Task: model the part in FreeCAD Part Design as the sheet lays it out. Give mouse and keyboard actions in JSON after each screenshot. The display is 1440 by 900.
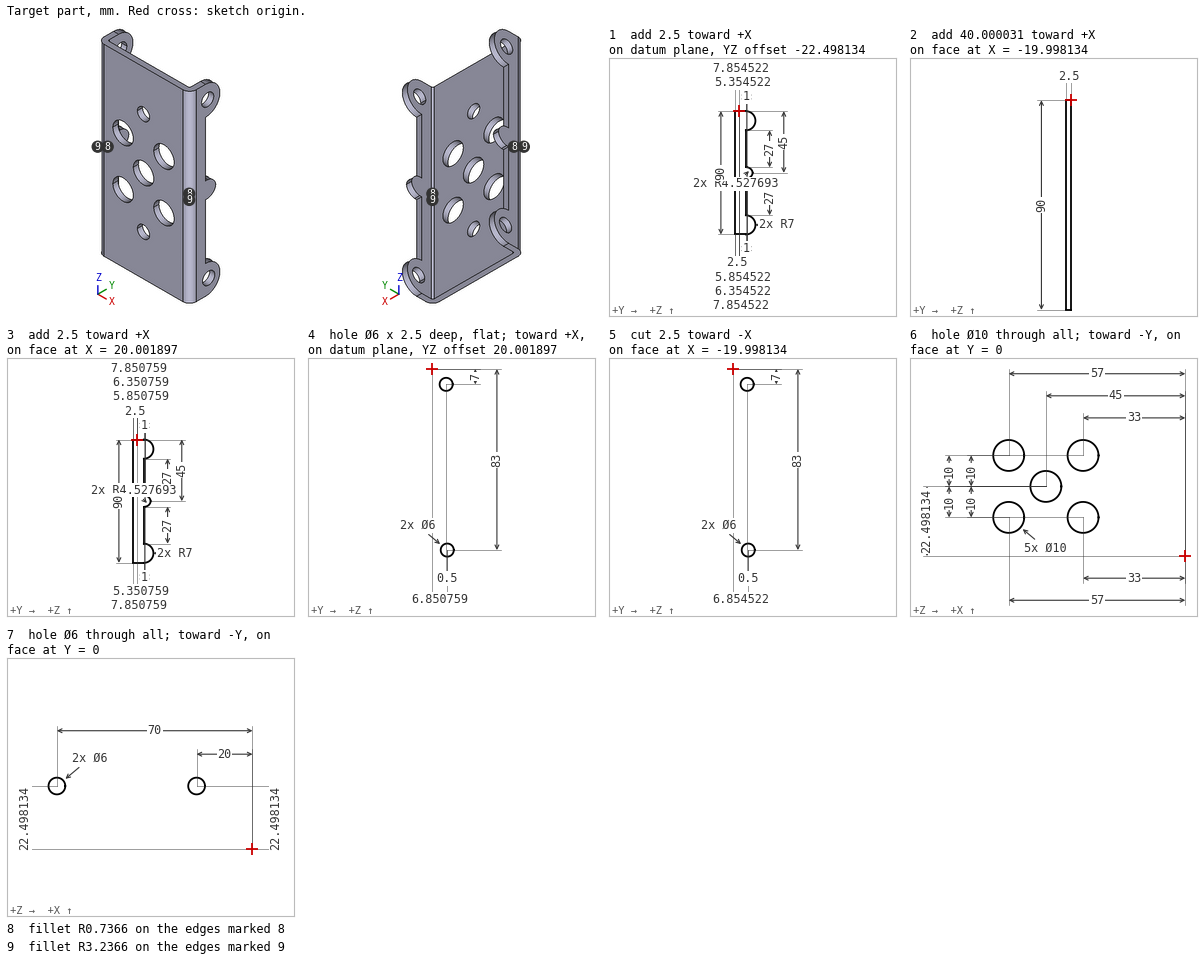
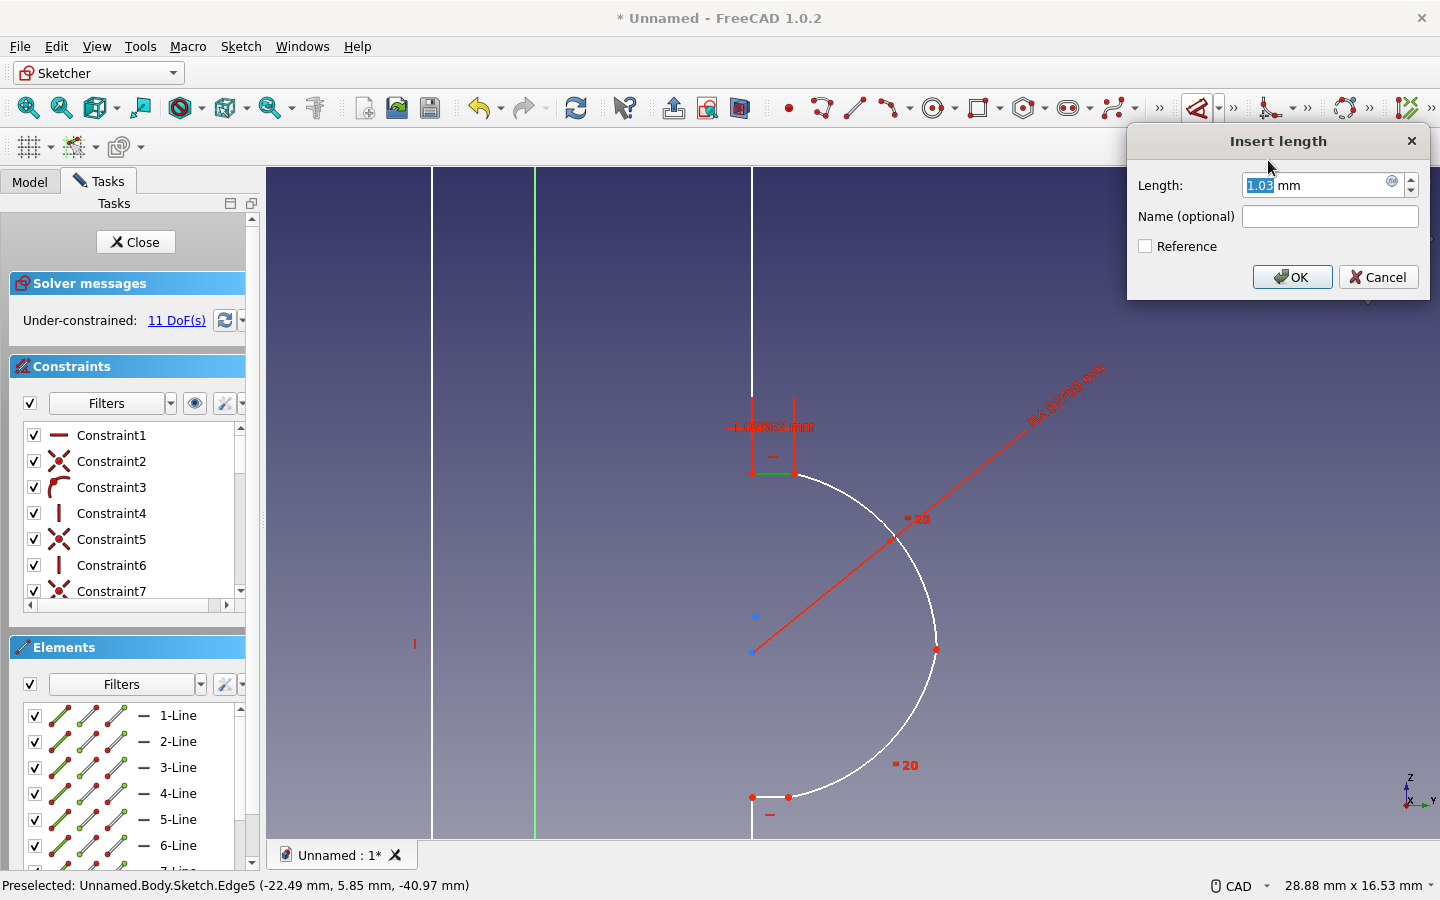
{"action": "type", "text": "1"}
{"action": "key", "text": "Return"}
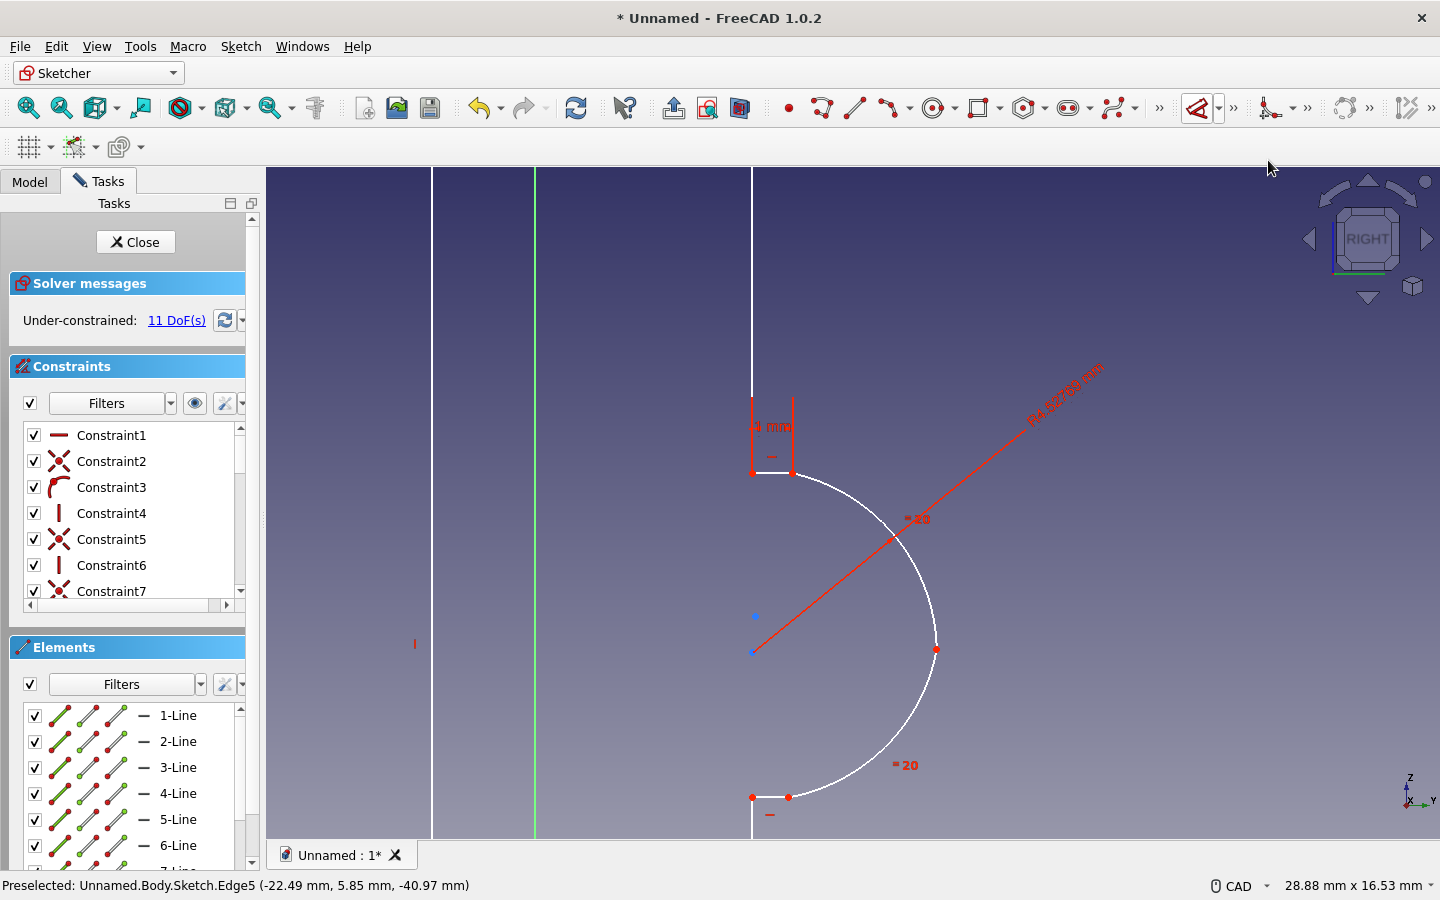
{"action": "scroll", "coordinate": [778, 797], "scroll_direction": "up", "scroll_amount": 2}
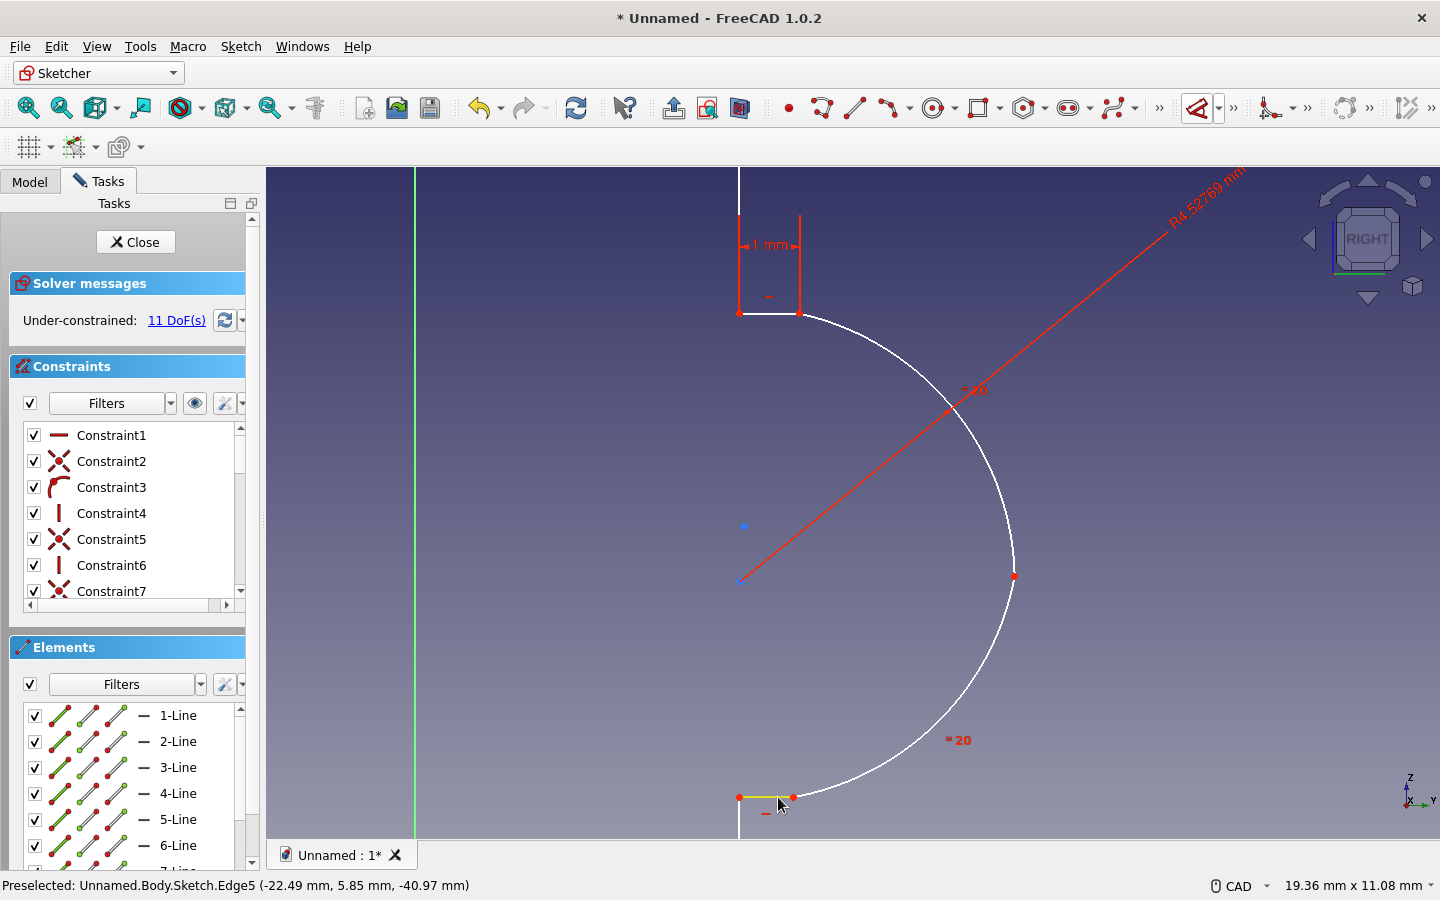
{"action": "left_click", "coordinate": [777, 797]}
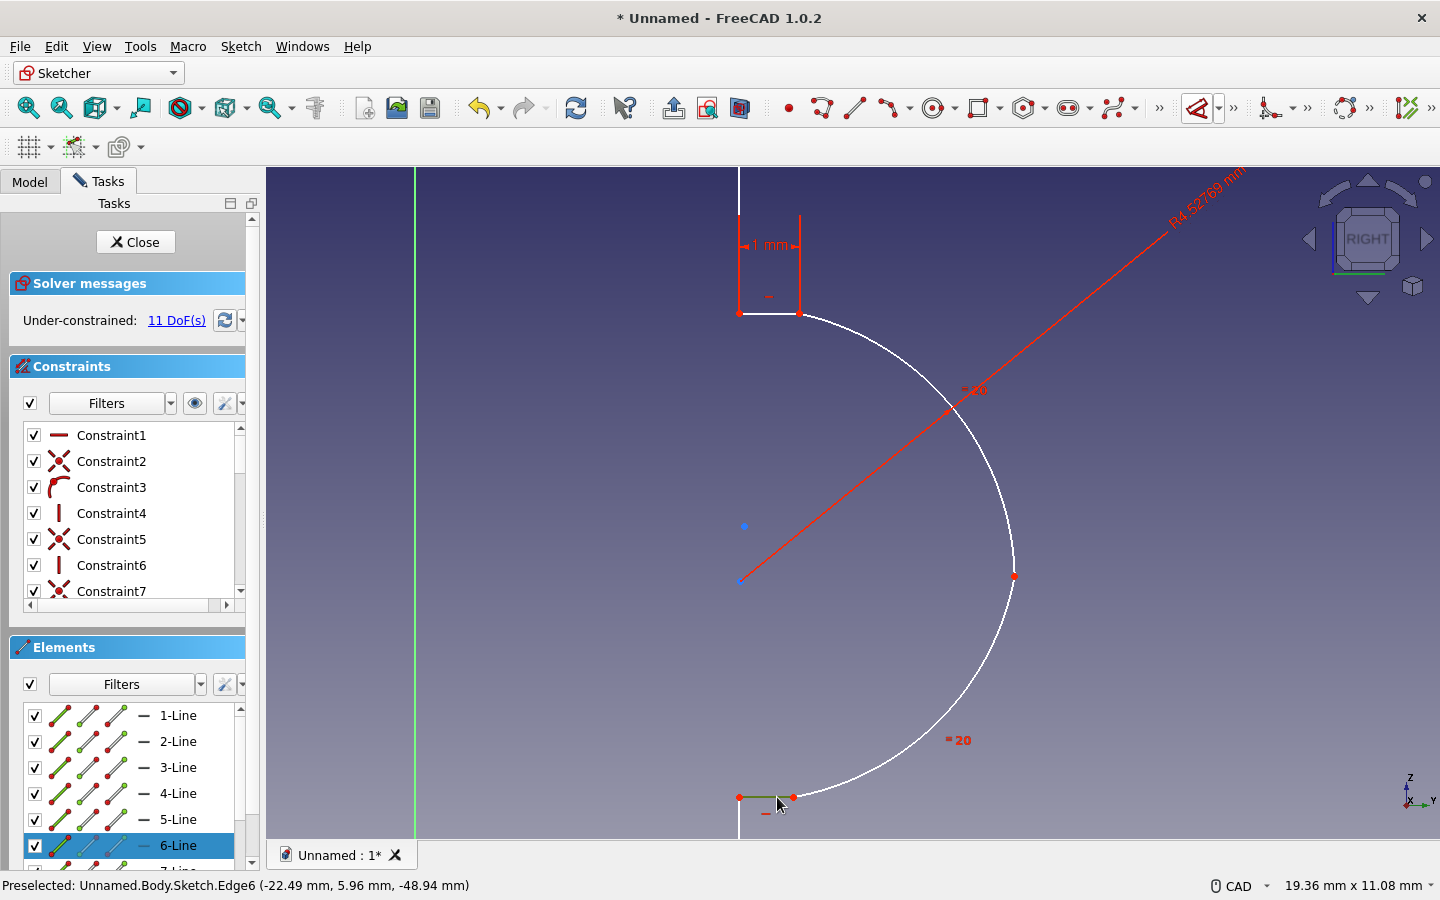
{"action": "left_click", "coordinate": [1218, 108]}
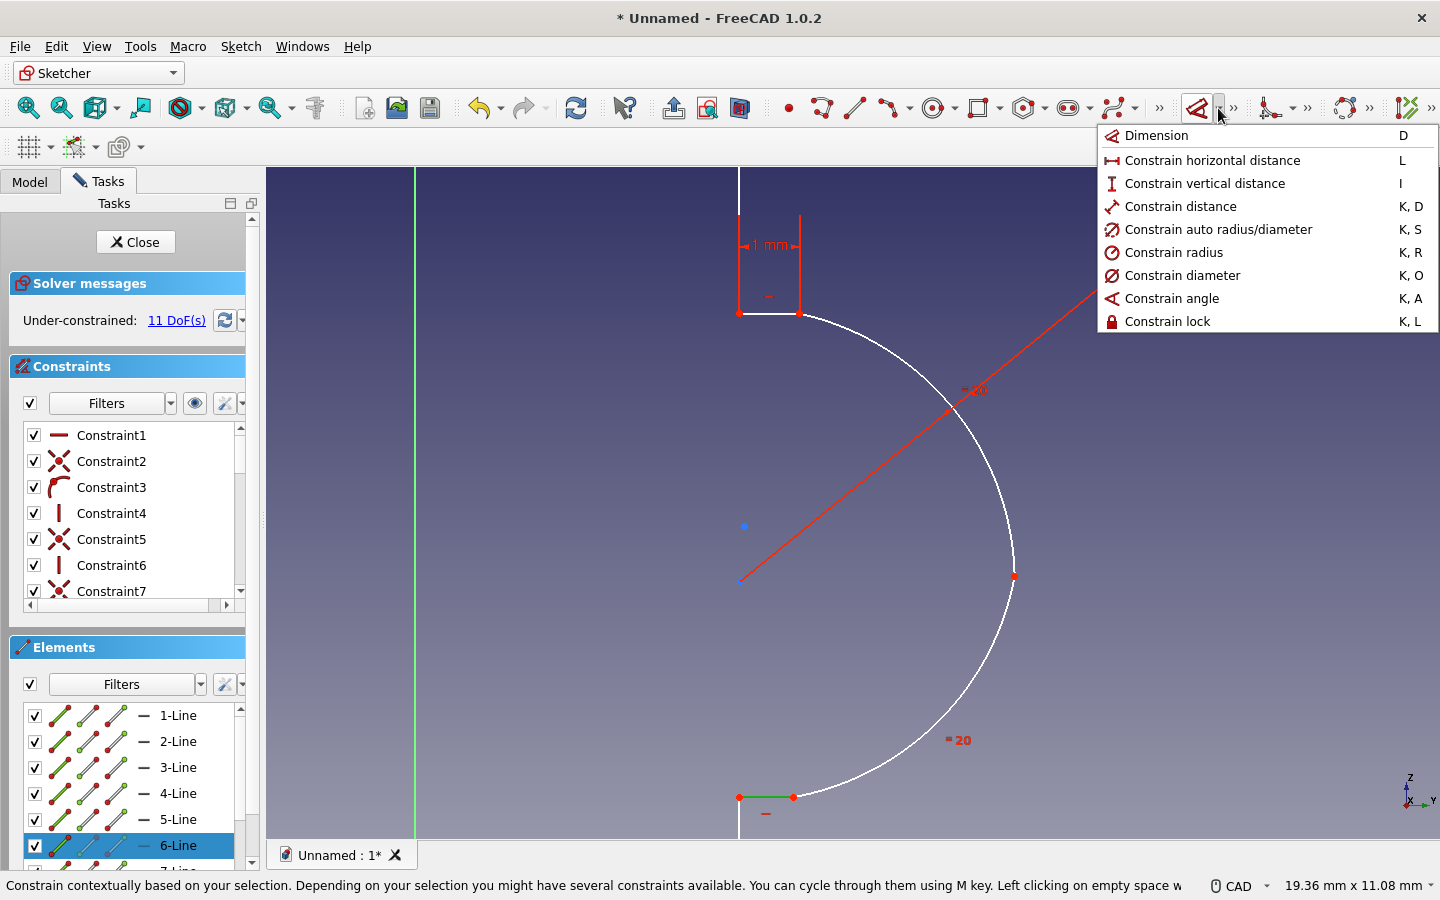
{"action": "left_click", "coordinate": [1268, 160]}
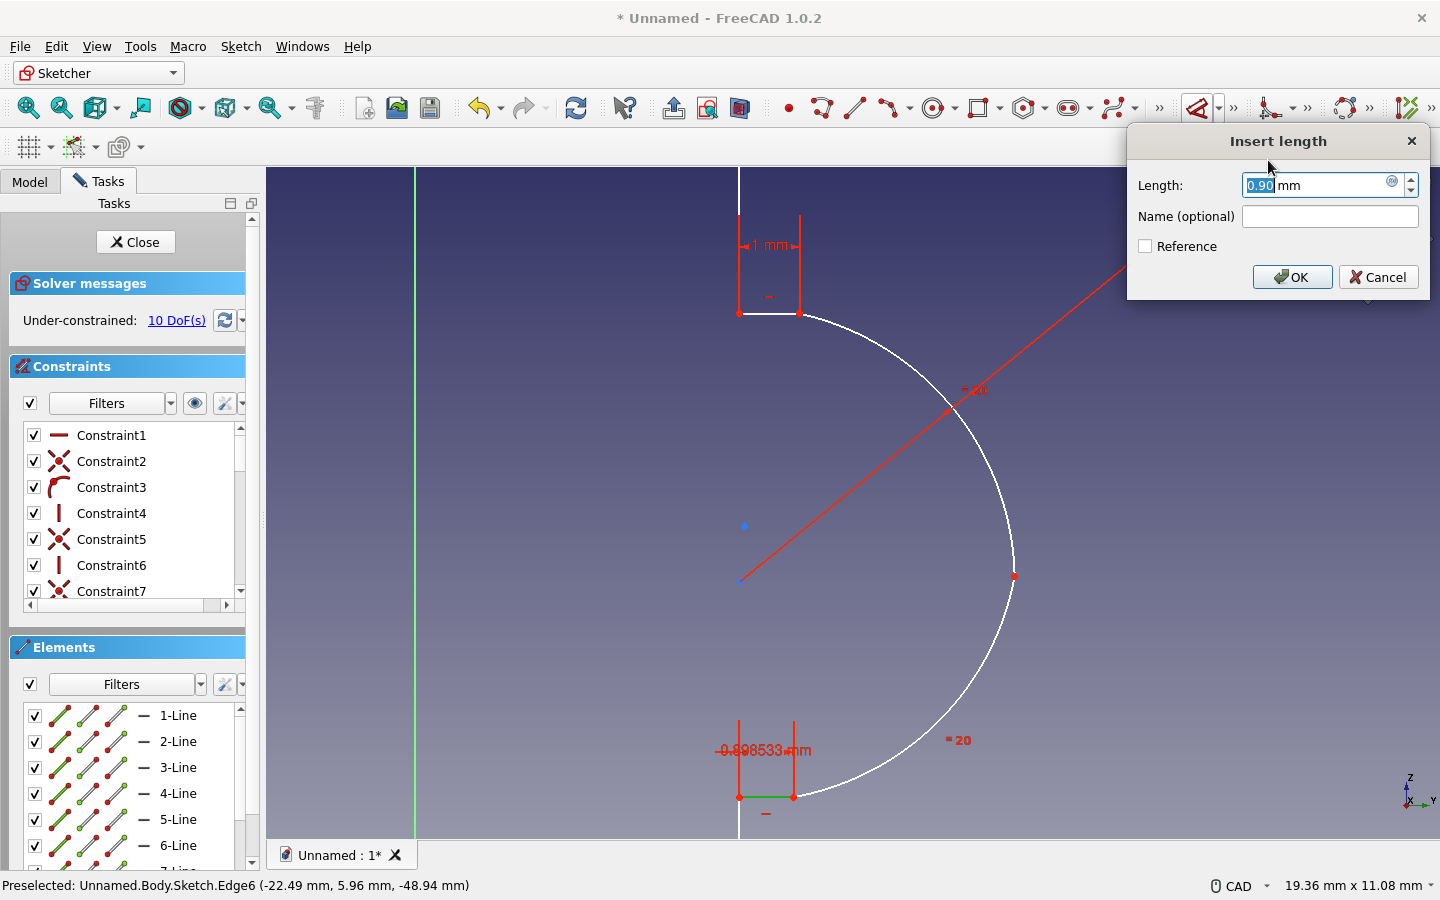
{"action": "type", "text": "1"}
{"action": "key", "text": "Return"}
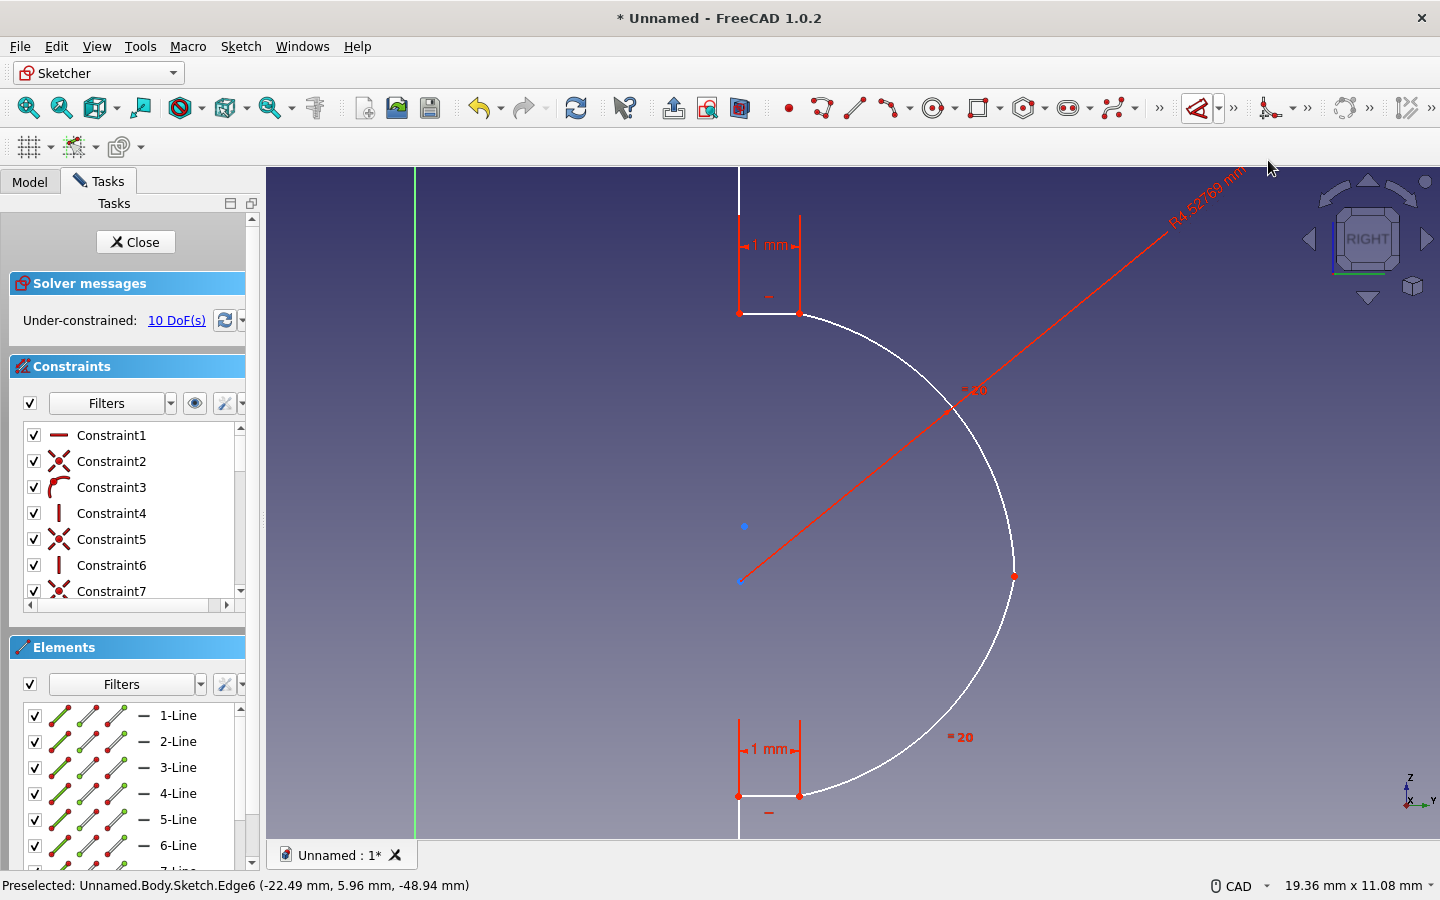
{"action": "scroll", "coordinate": [790, 499], "scroll_direction": "down", "scroll_amount": 13}